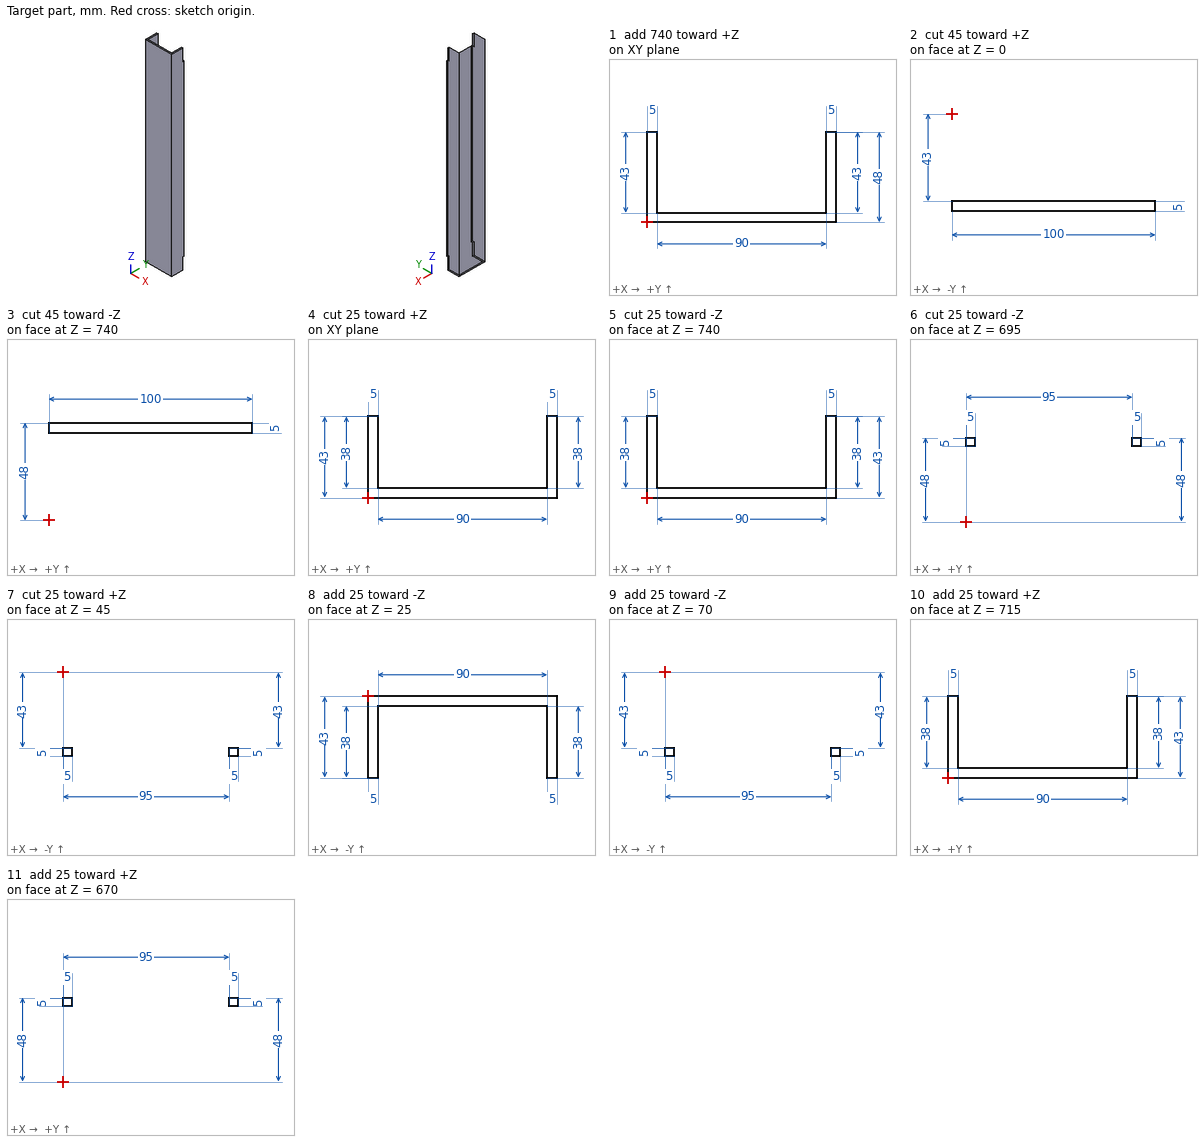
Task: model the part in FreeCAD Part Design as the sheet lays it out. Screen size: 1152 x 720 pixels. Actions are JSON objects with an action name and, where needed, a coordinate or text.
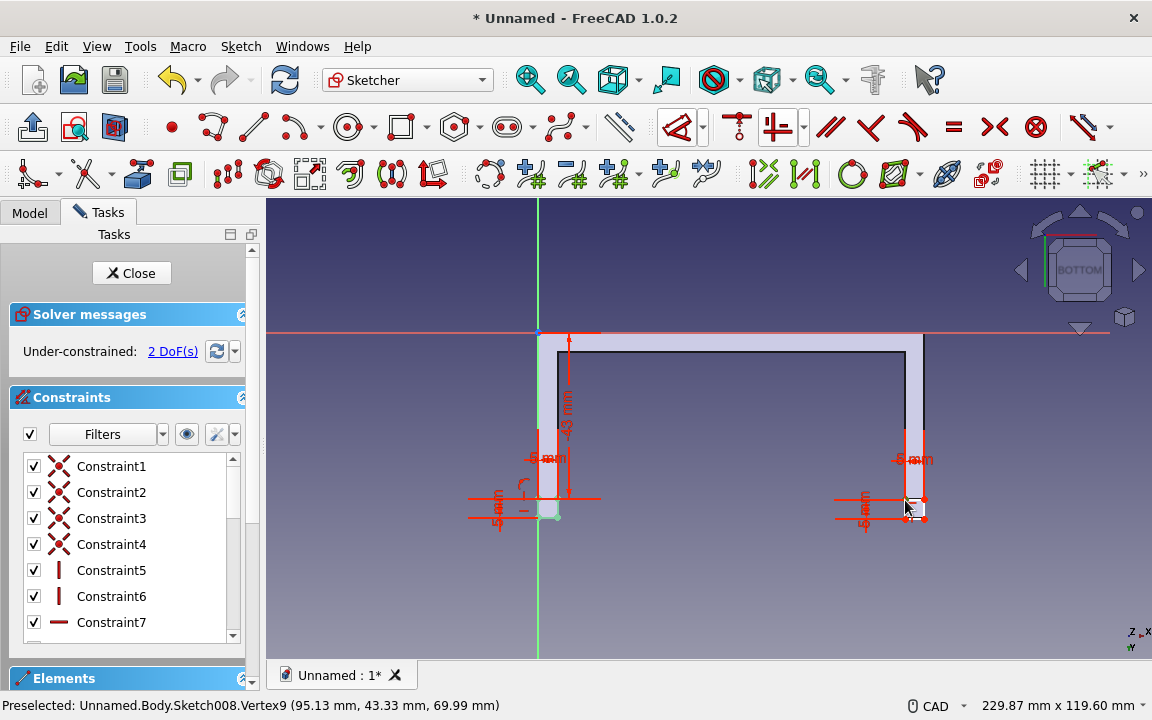
{"action": "key", "text": "l"}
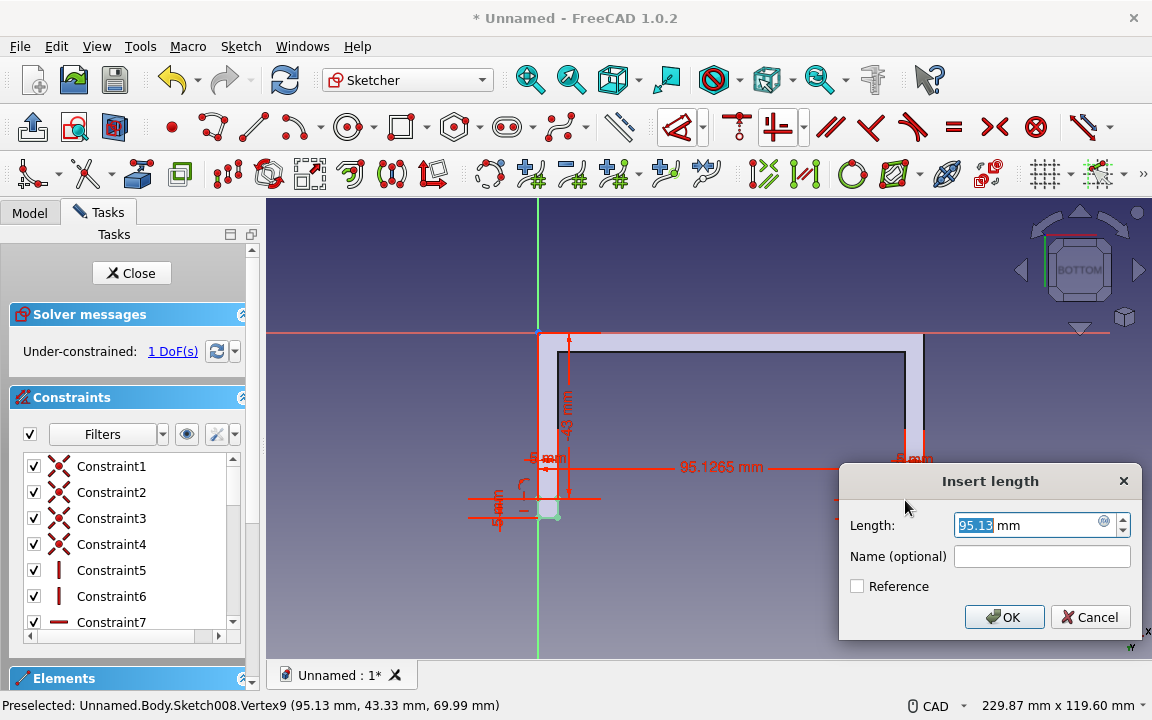
{"action": "type", "text": "95"}
{"action": "key", "text": "Return"}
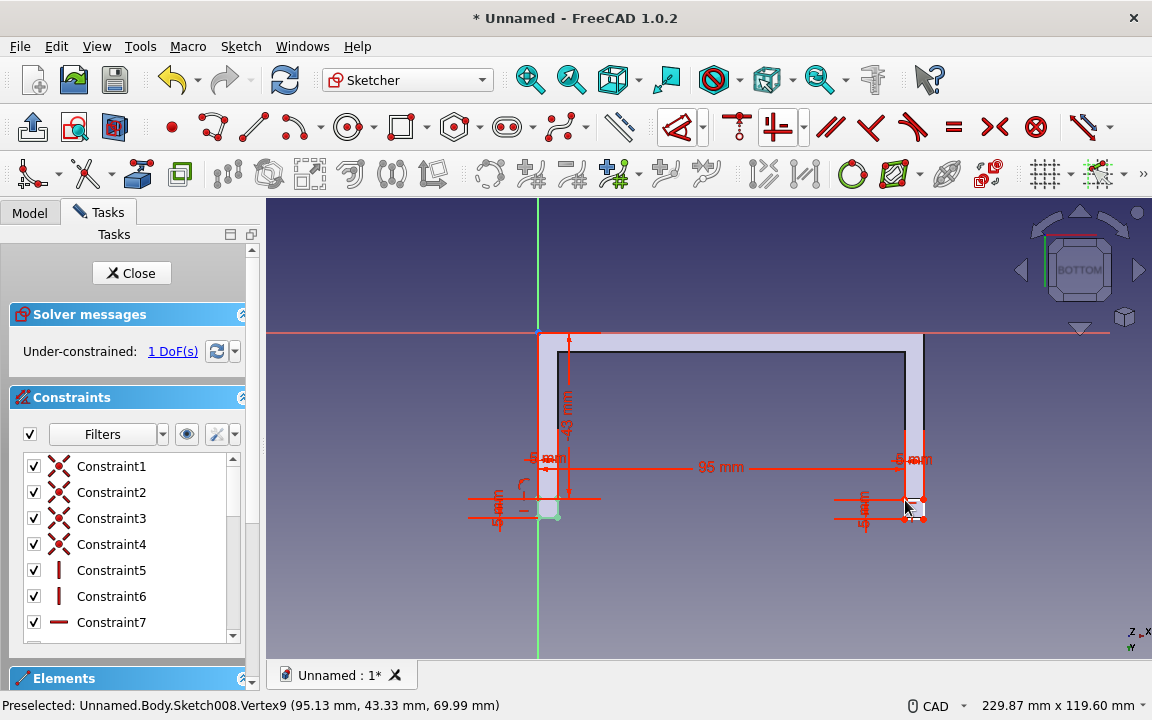
{"action": "left_click", "coordinate": [905, 500]}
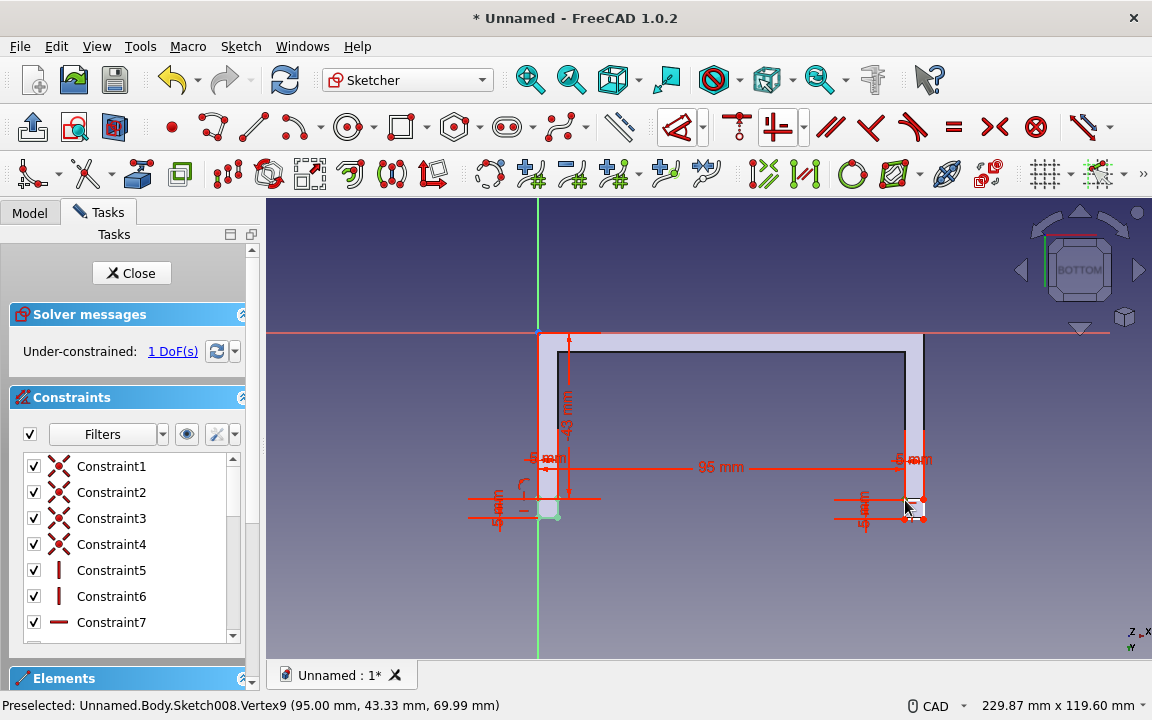
{"action": "left_click", "coordinate": [702, 128]}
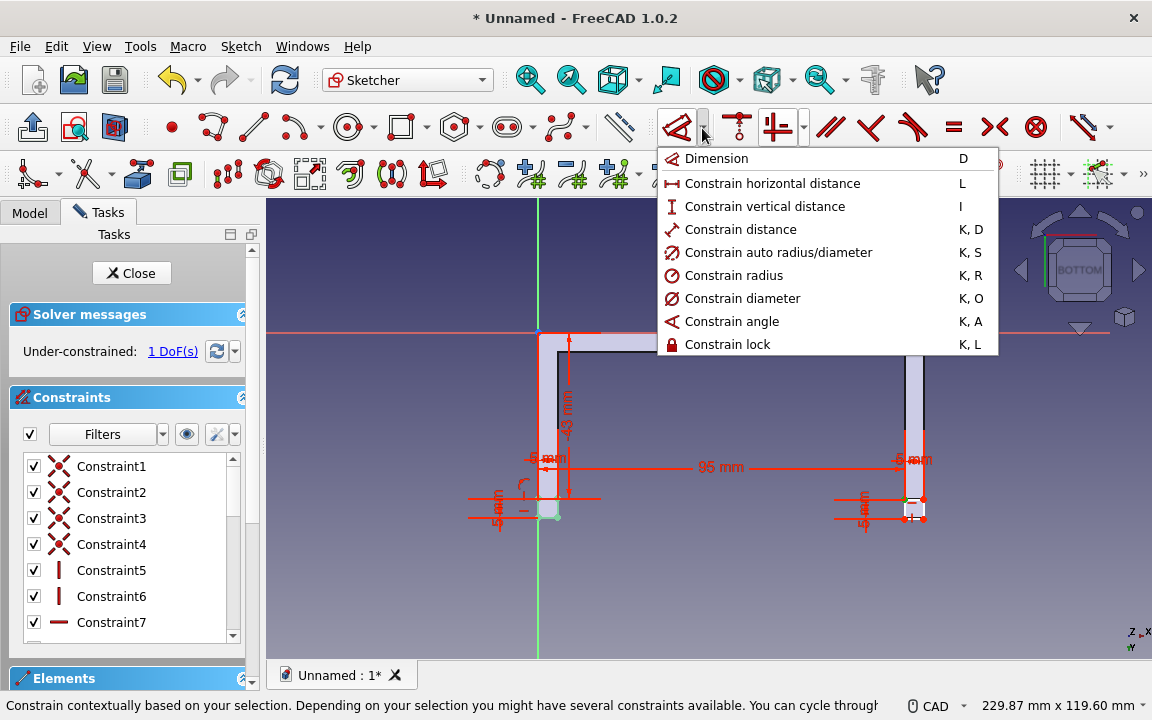
{"action": "left_click", "coordinate": [828, 206]}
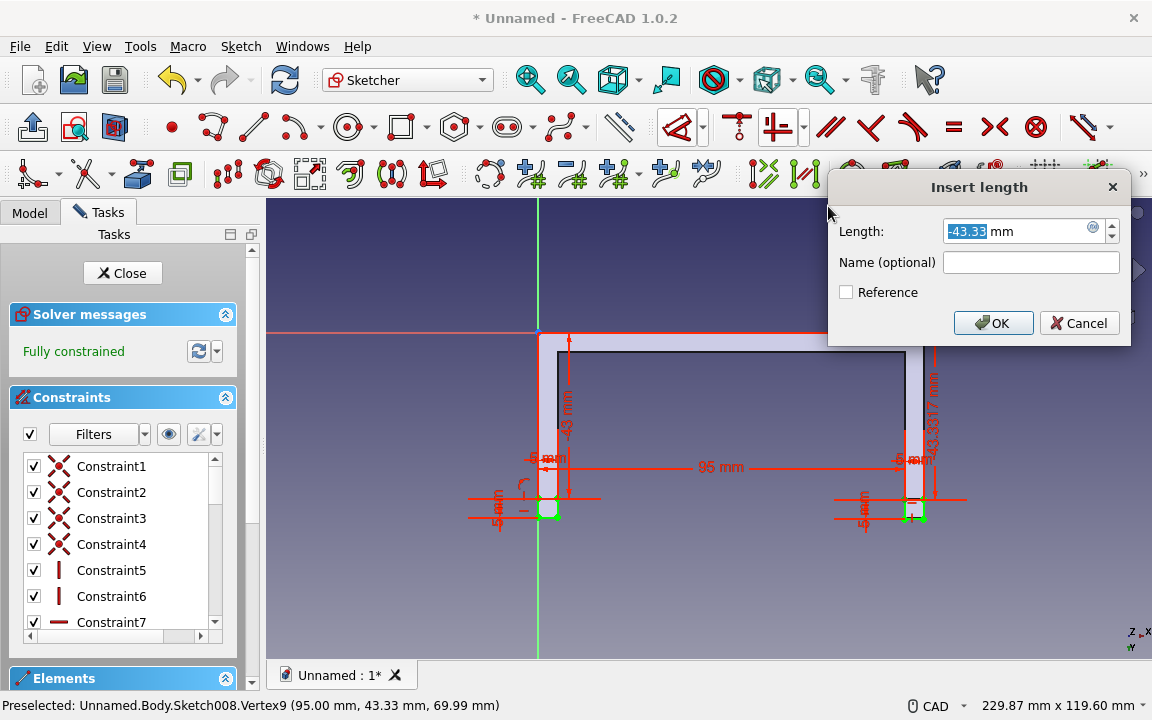
{"action": "type", "text": "-43"}
{"action": "key", "text": "Return"}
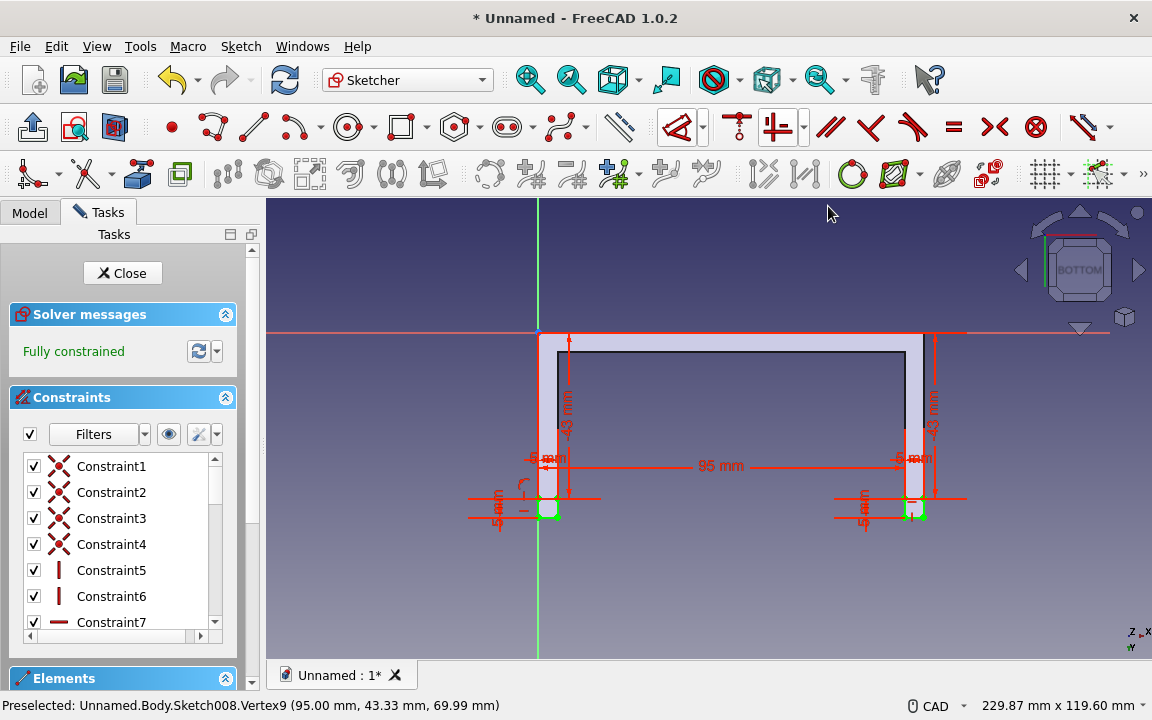
{"action": "left_click", "coordinate": [123, 273]}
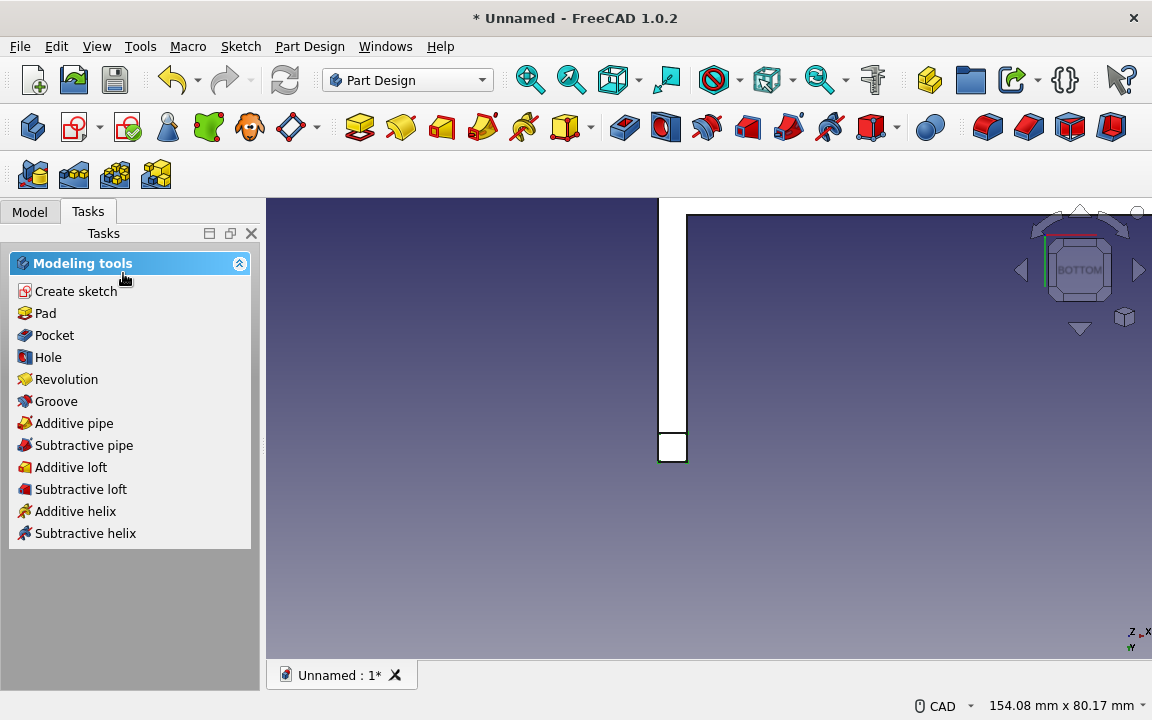
{"action": "left_click", "coordinate": [360, 128]}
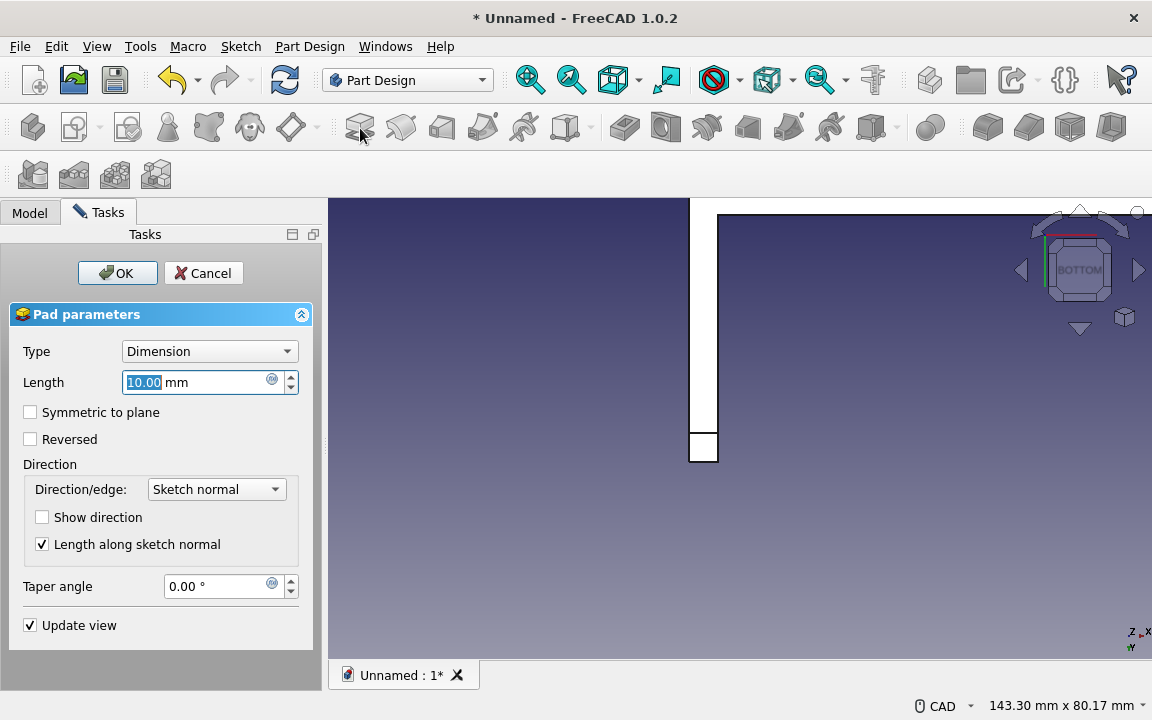
{"action": "type", "text": "25"}
{"action": "key", "text": "Tab"}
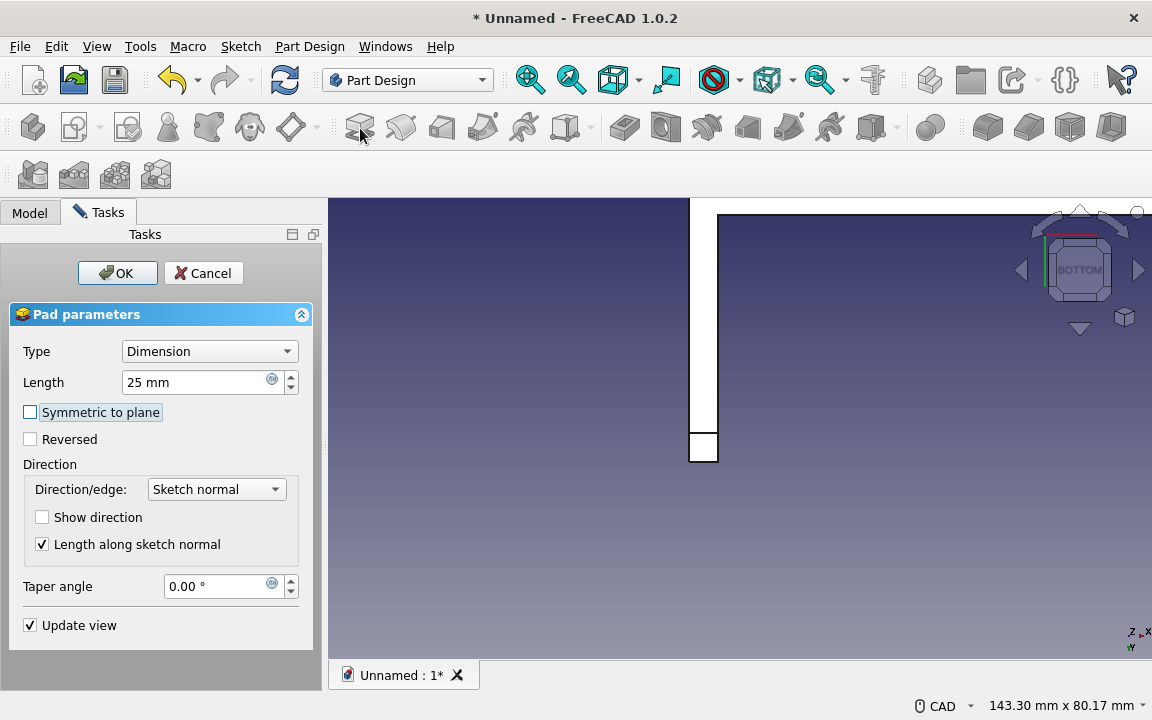
{"action": "left_click", "coordinate": [118, 273]}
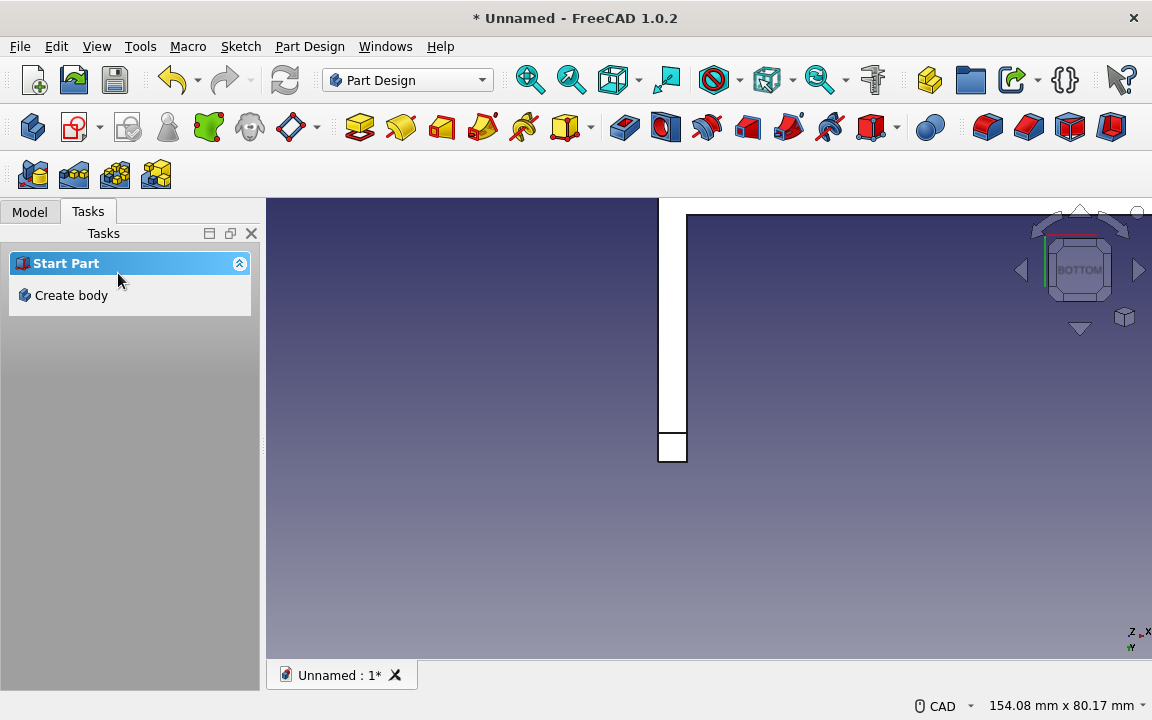
{"action": "key", "text": "v f"}